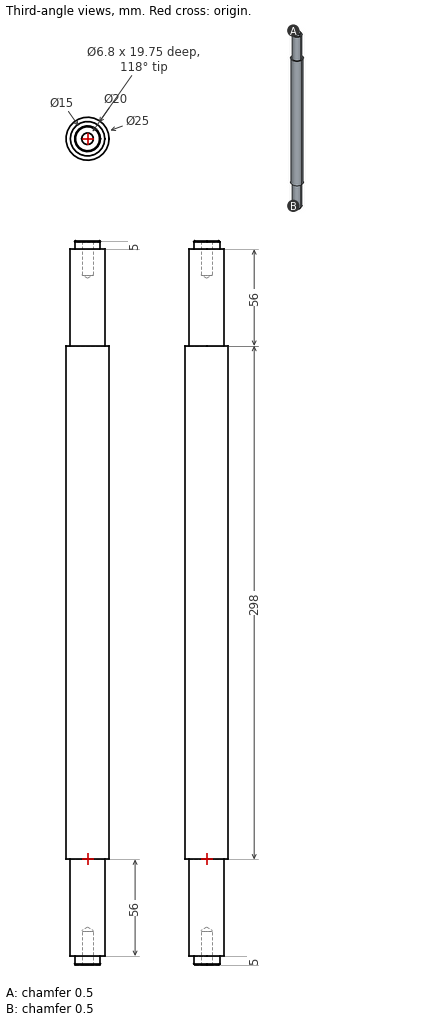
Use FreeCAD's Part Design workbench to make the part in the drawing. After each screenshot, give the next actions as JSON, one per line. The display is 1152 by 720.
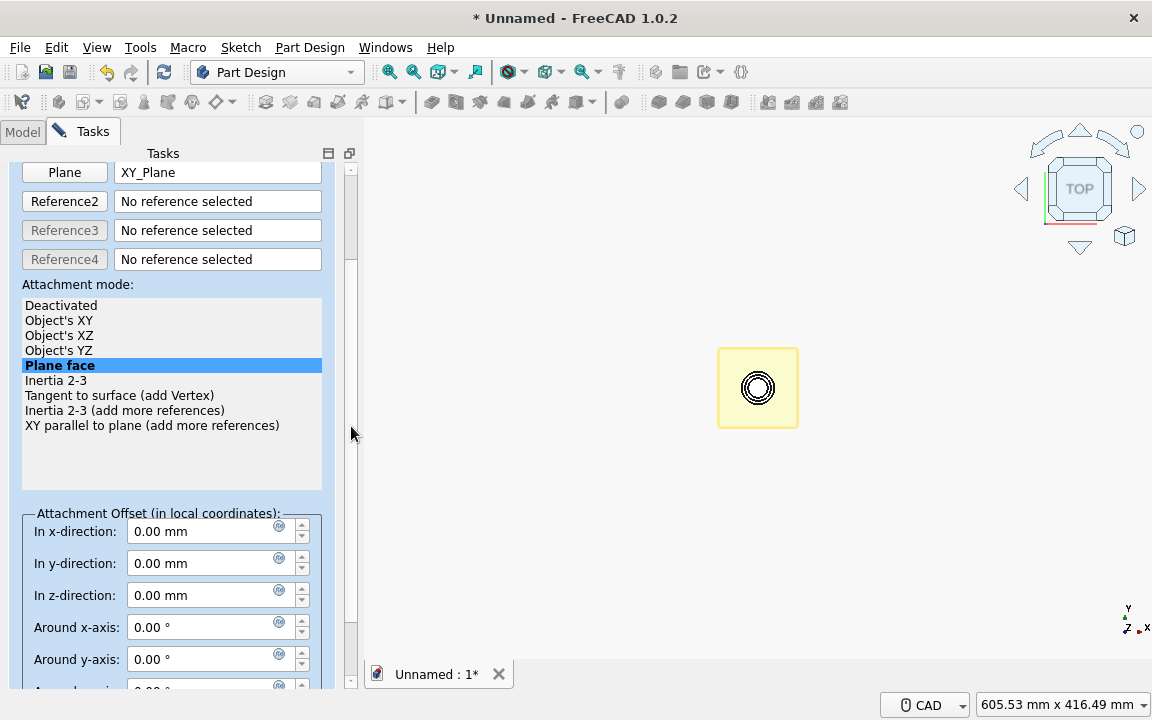
{"action": "triple_click", "coordinate": [210, 595]}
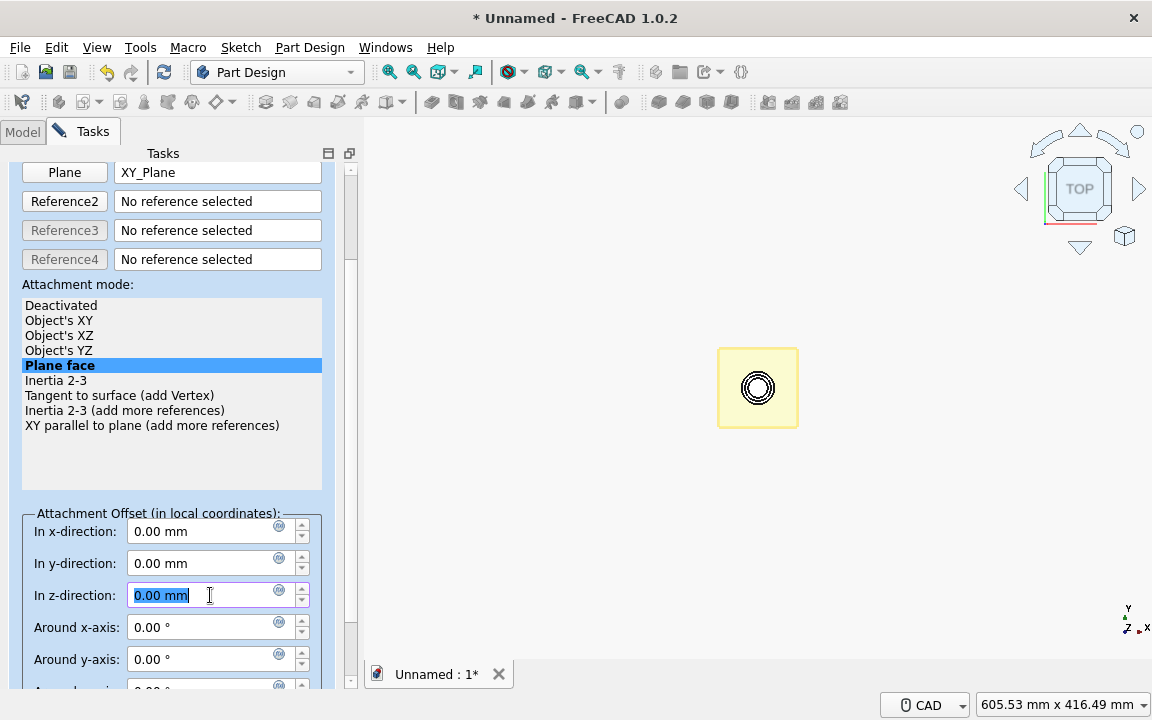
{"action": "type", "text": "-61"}
{"action": "key", "text": "Tab"}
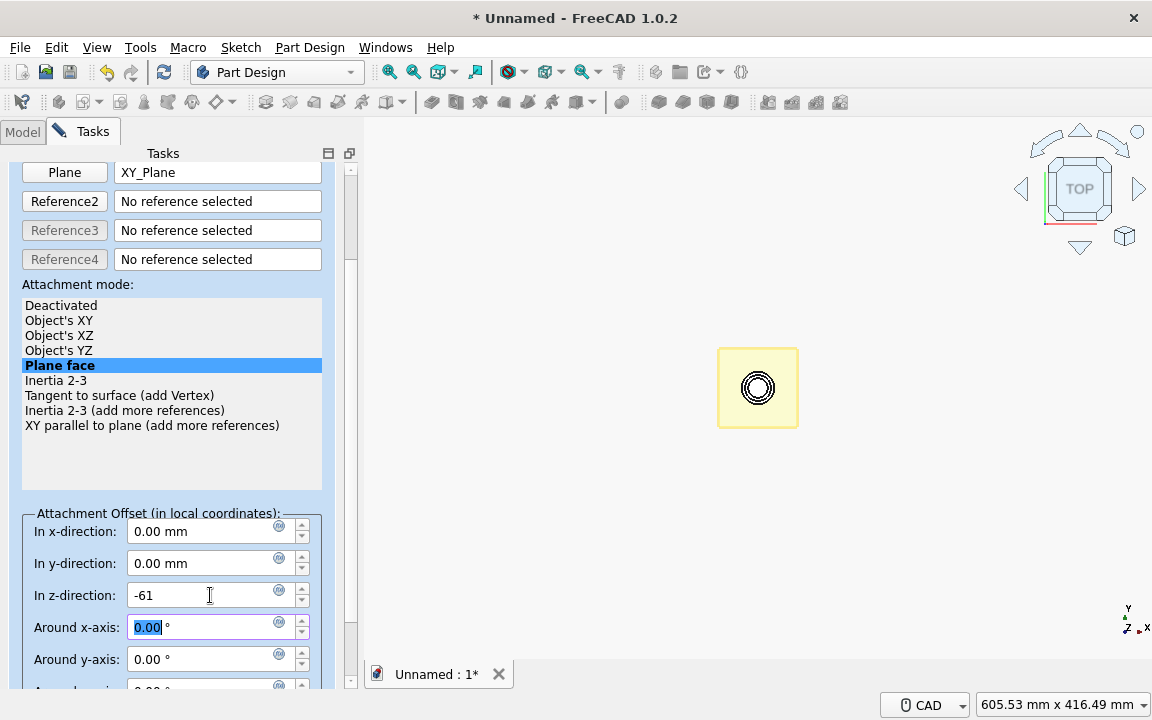
{"action": "scroll", "coordinate": [351, 426], "scroll_direction": "up", "scroll_amount": 3}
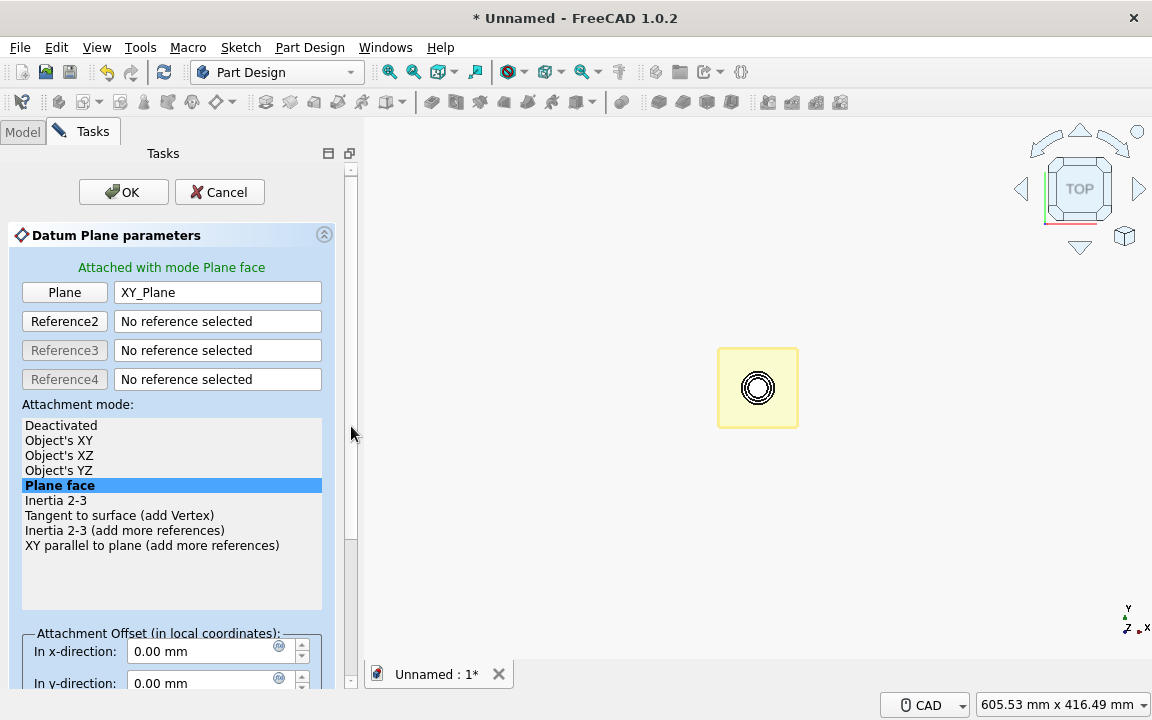
{"action": "left_click", "coordinate": [124, 192]}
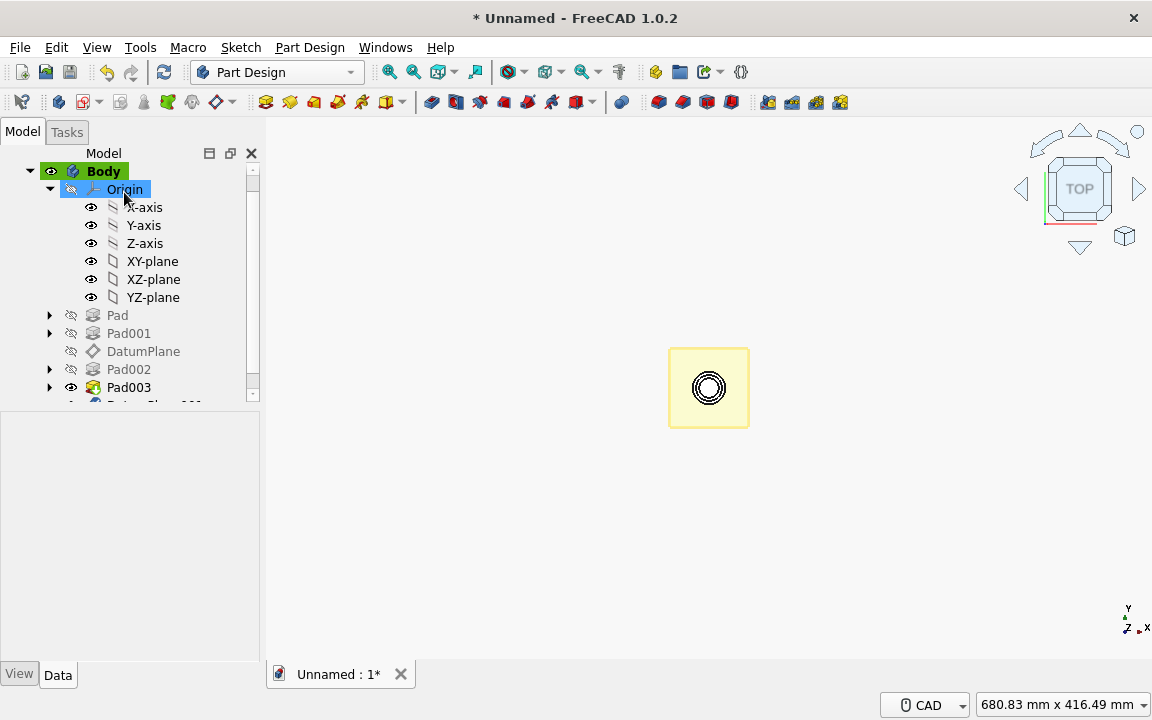
{"action": "scroll", "coordinate": [120, 275], "scroll_direction": "down", "scroll_amount": 3}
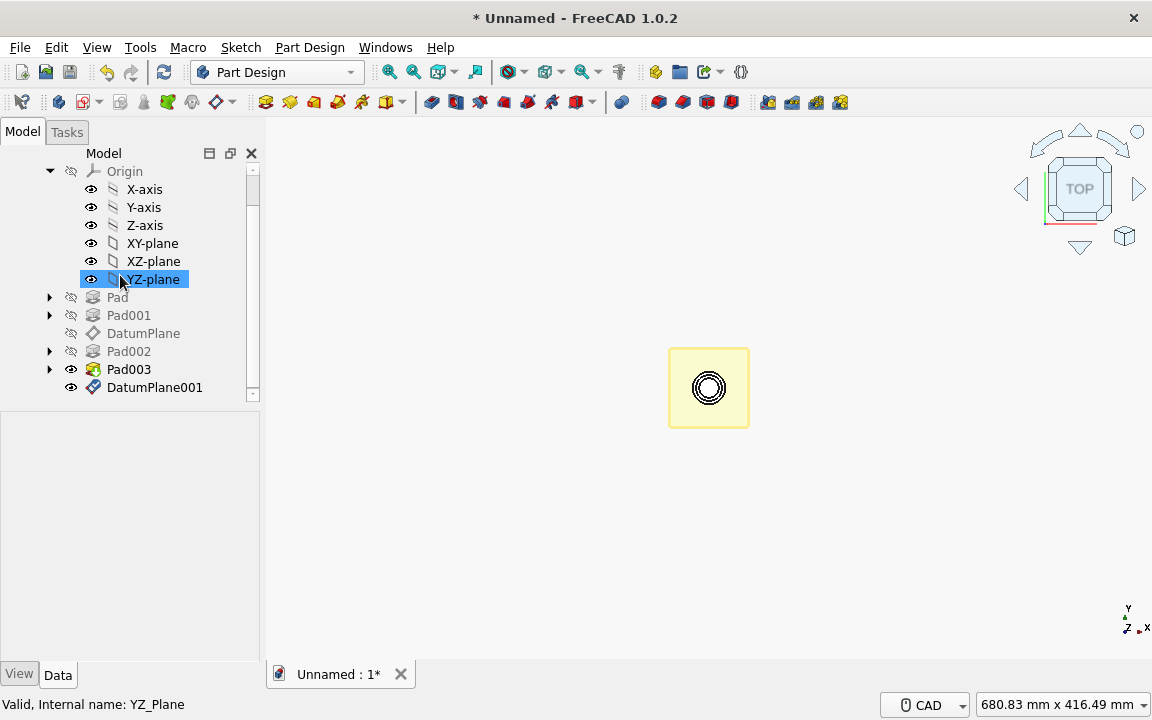
{"action": "left_click", "coordinate": [116, 387]}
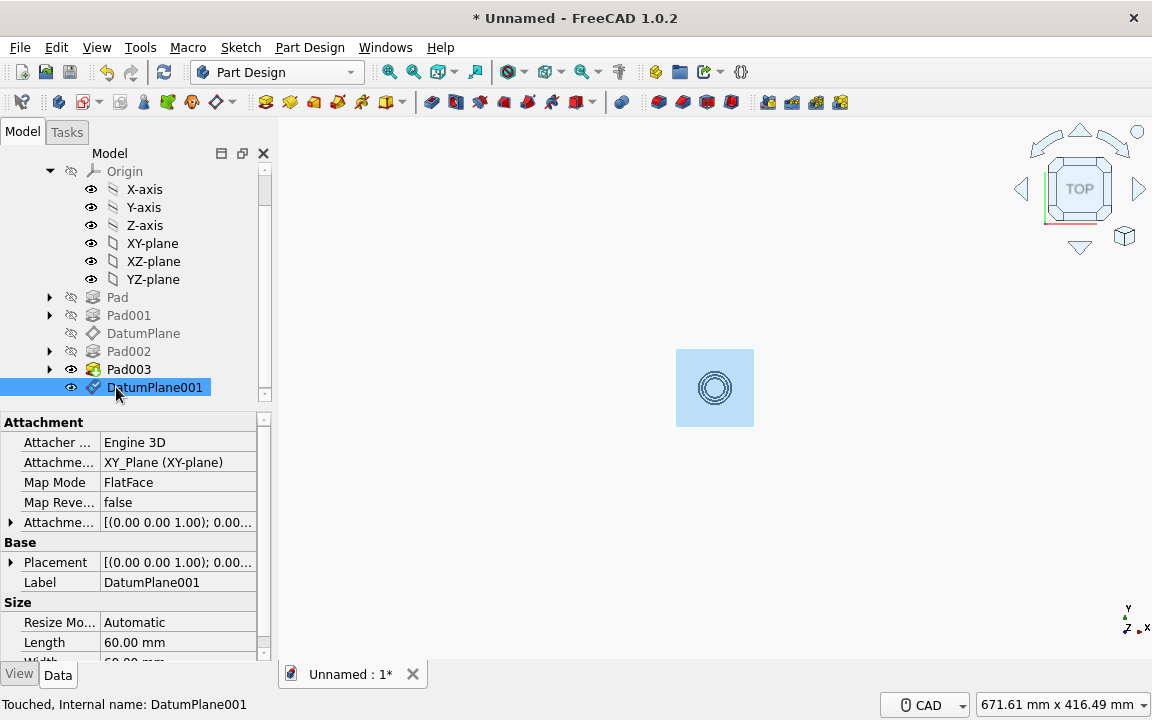
{"action": "left_click", "coordinate": [84, 102]}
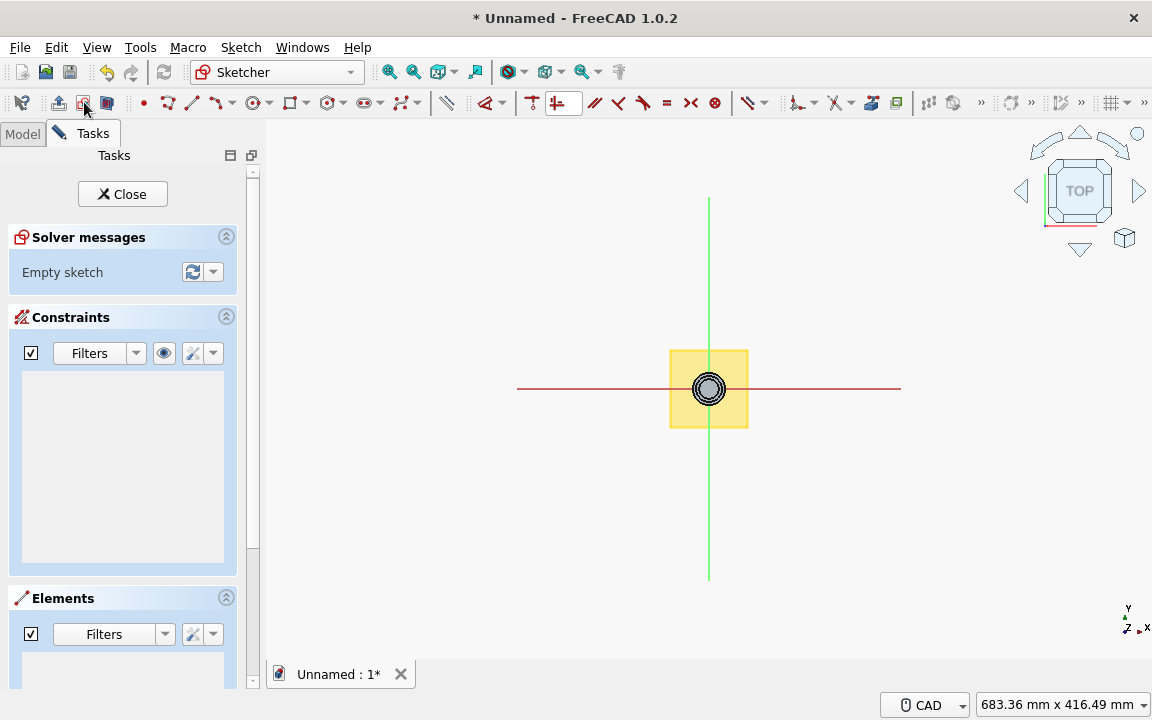
{"action": "left_click", "coordinate": [108, 104]}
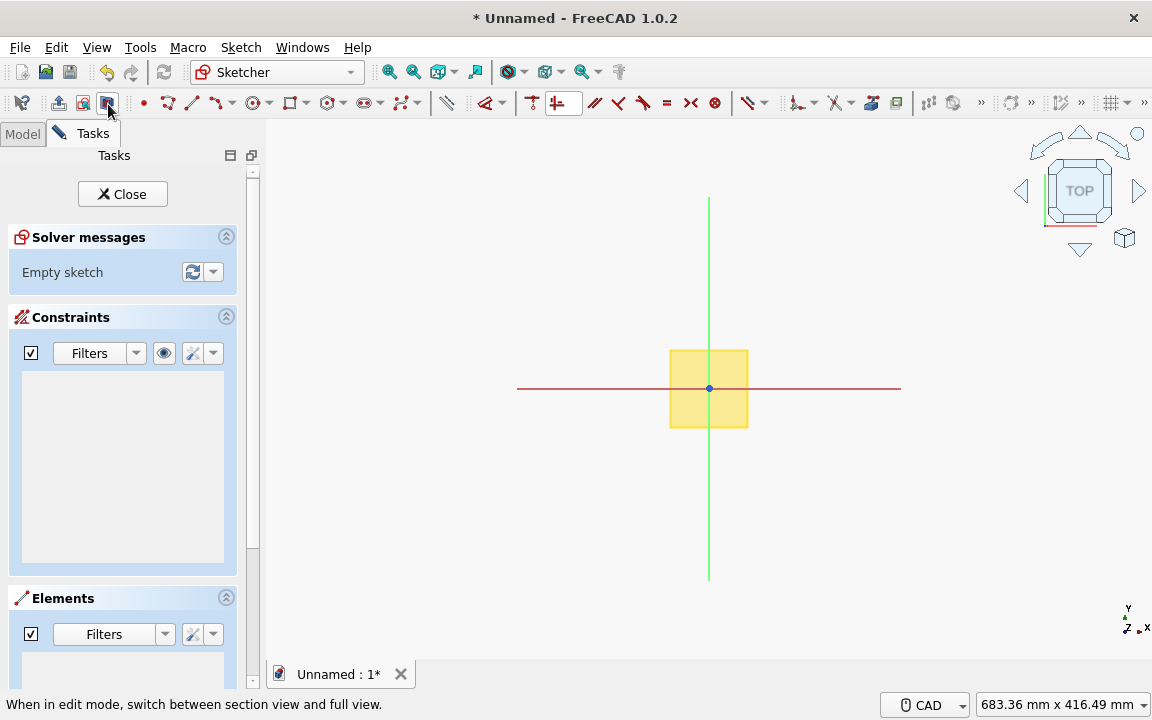
{"action": "scroll", "coordinate": [713, 389], "scroll_direction": "up", "scroll_amount": 14}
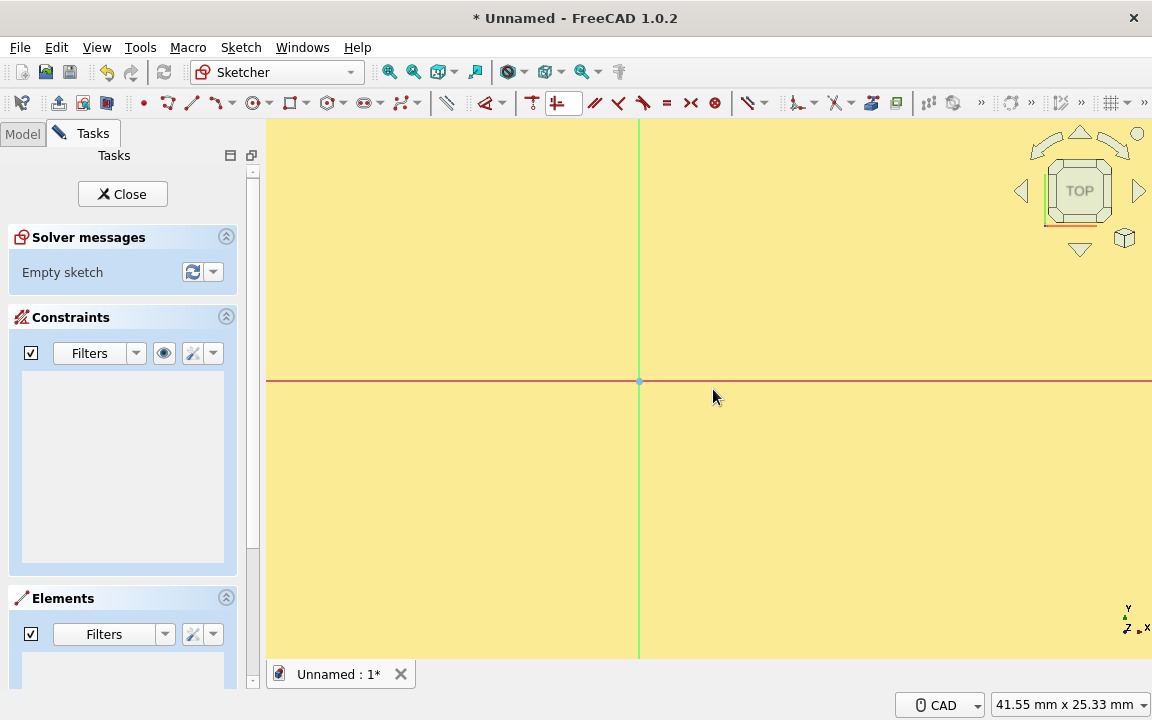
{"action": "left_click", "coordinate": [254, 104]}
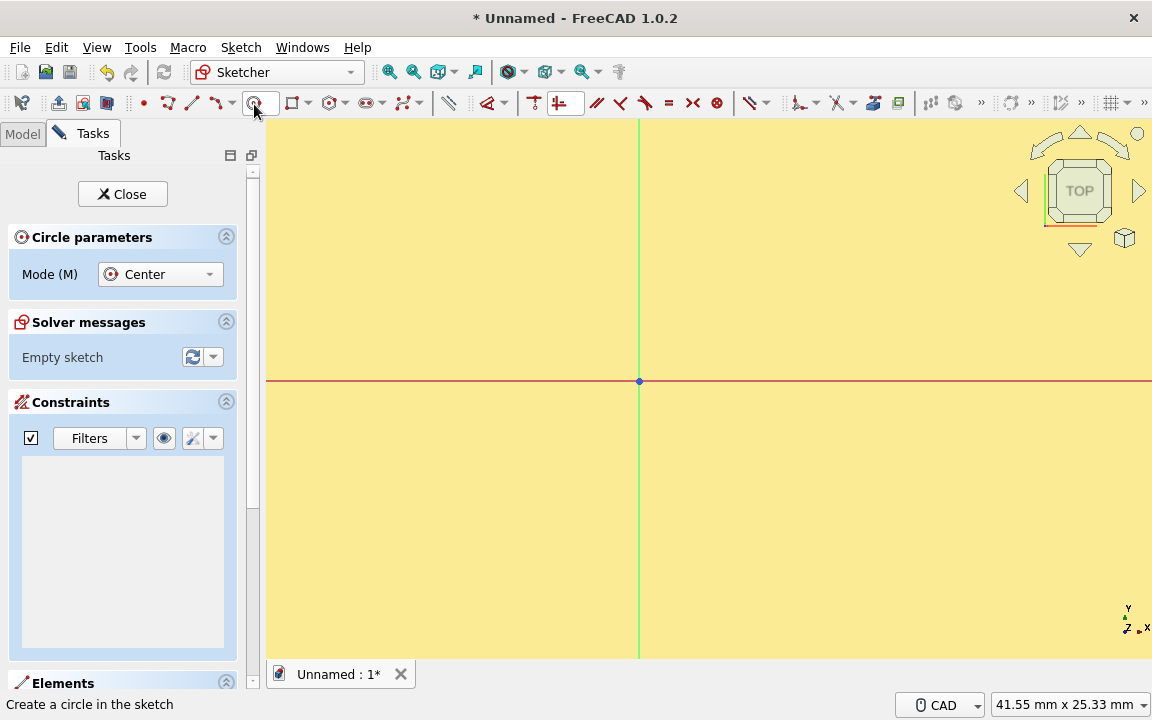
{"action": "left_click", "coordinate": [639, 381]}
{"action": "left_click", "coordinate": [752, 268]}
{"action": "key", "text": "Escape"}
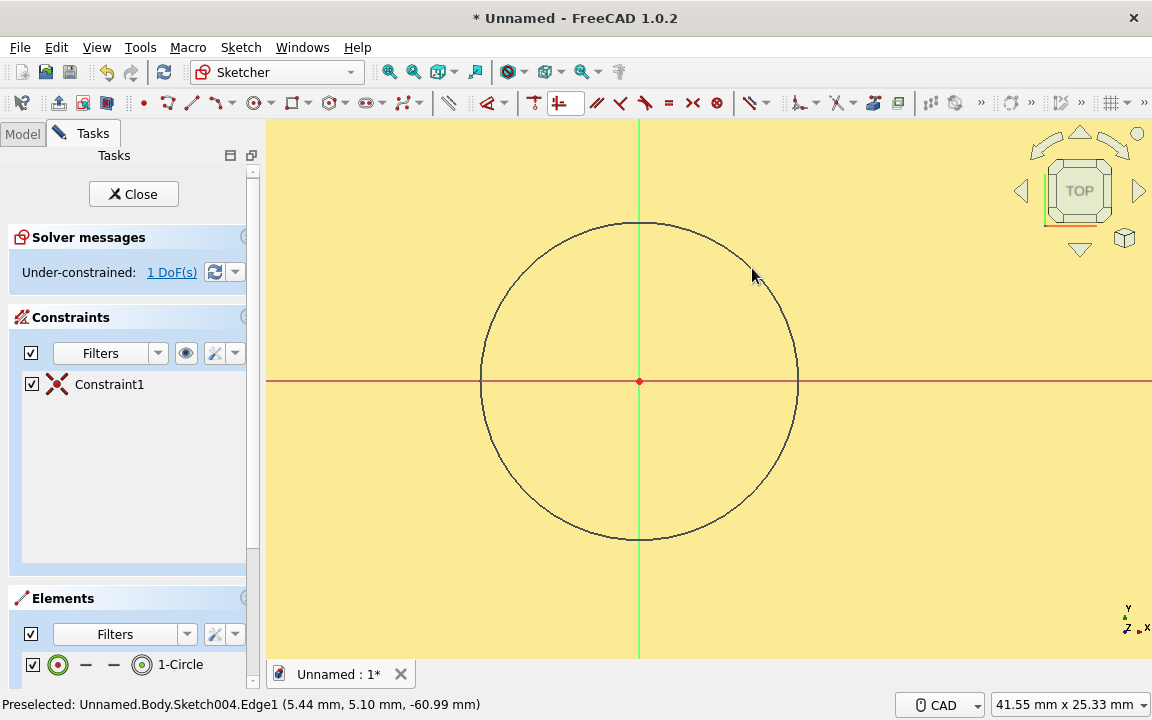
{"action": "left_click", "coordinate": [488, 104]}